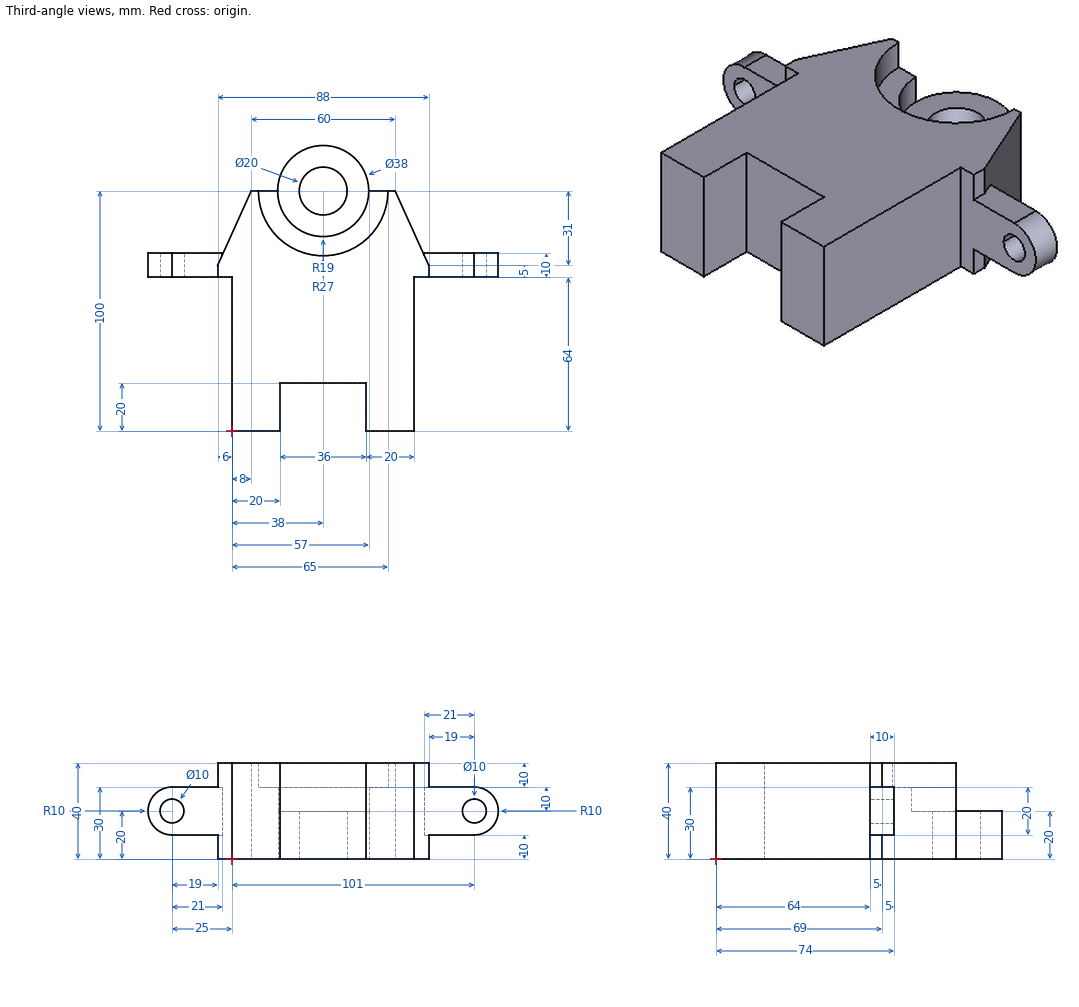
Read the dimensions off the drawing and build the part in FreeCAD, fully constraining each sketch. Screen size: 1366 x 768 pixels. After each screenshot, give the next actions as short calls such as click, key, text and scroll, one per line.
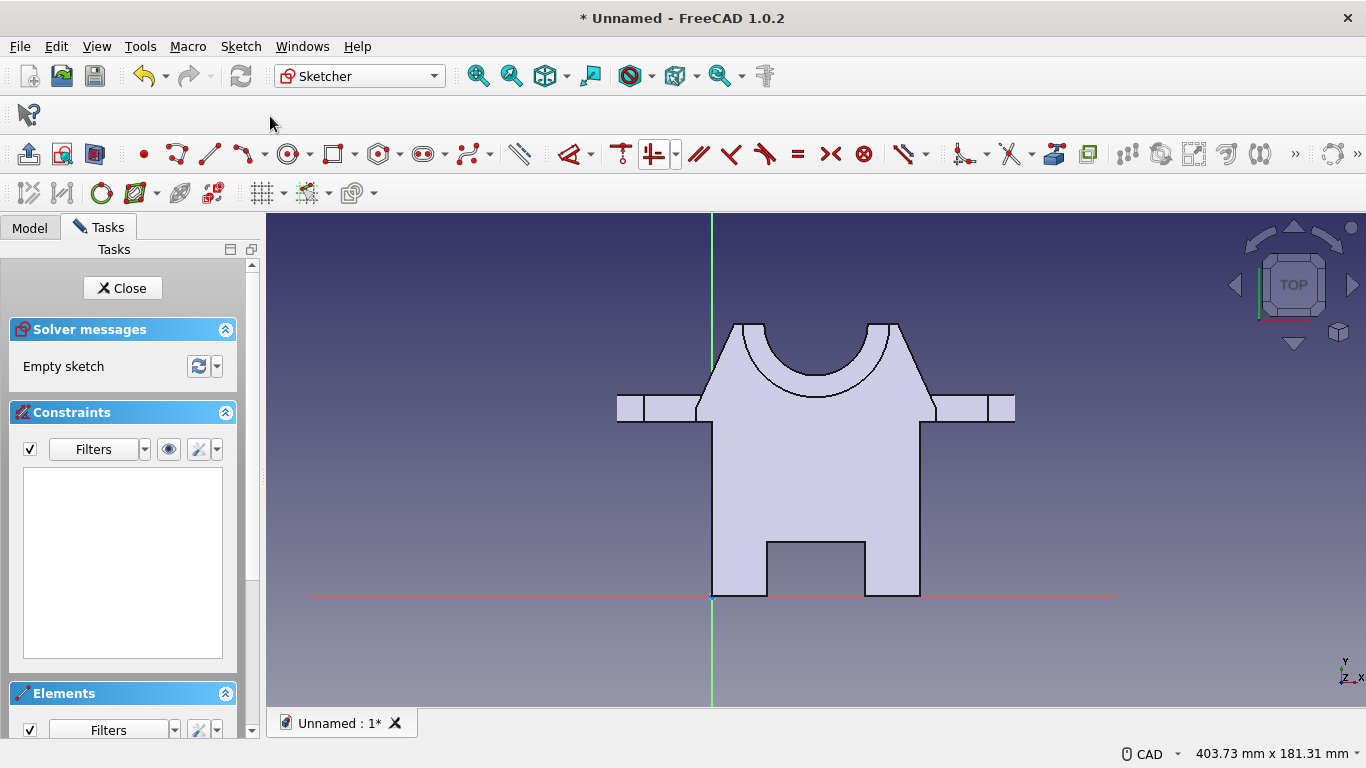
click(95, 154)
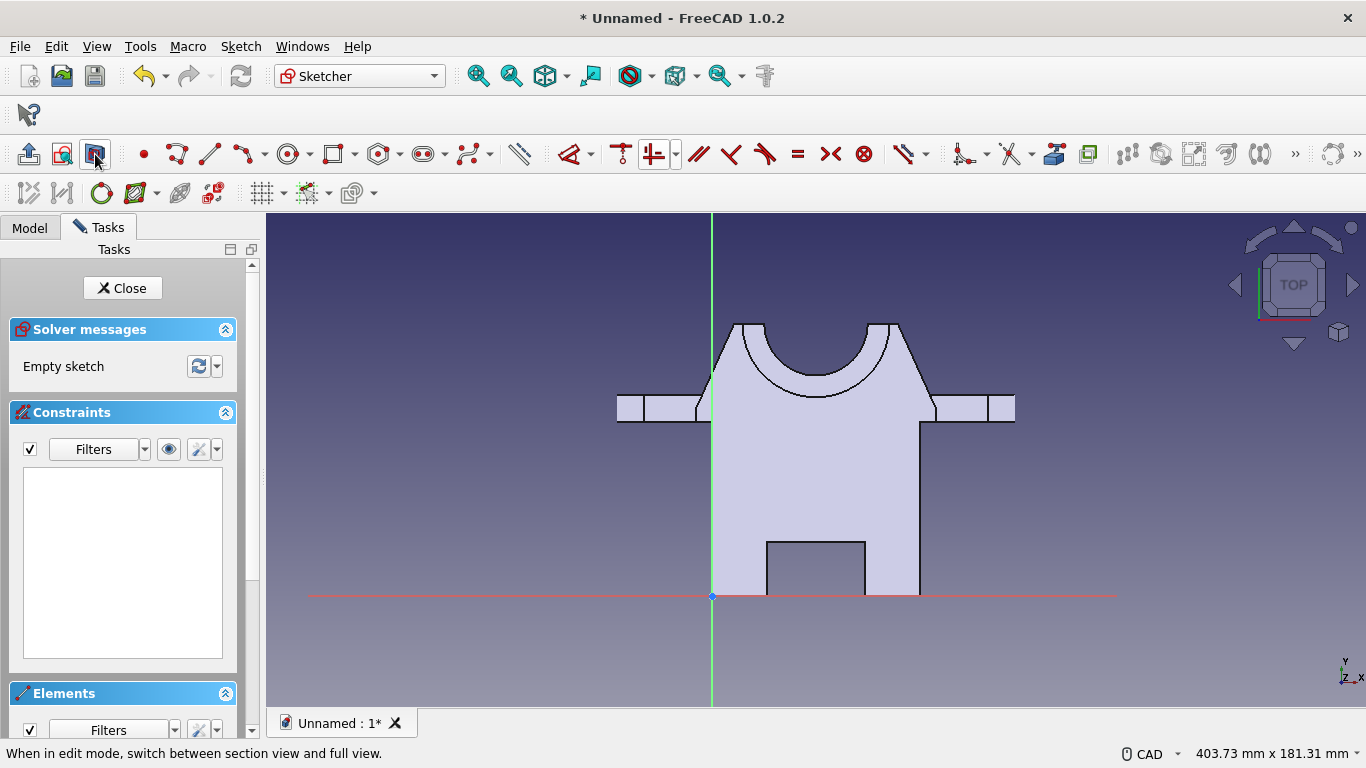
scroll(856, 244, up, 5)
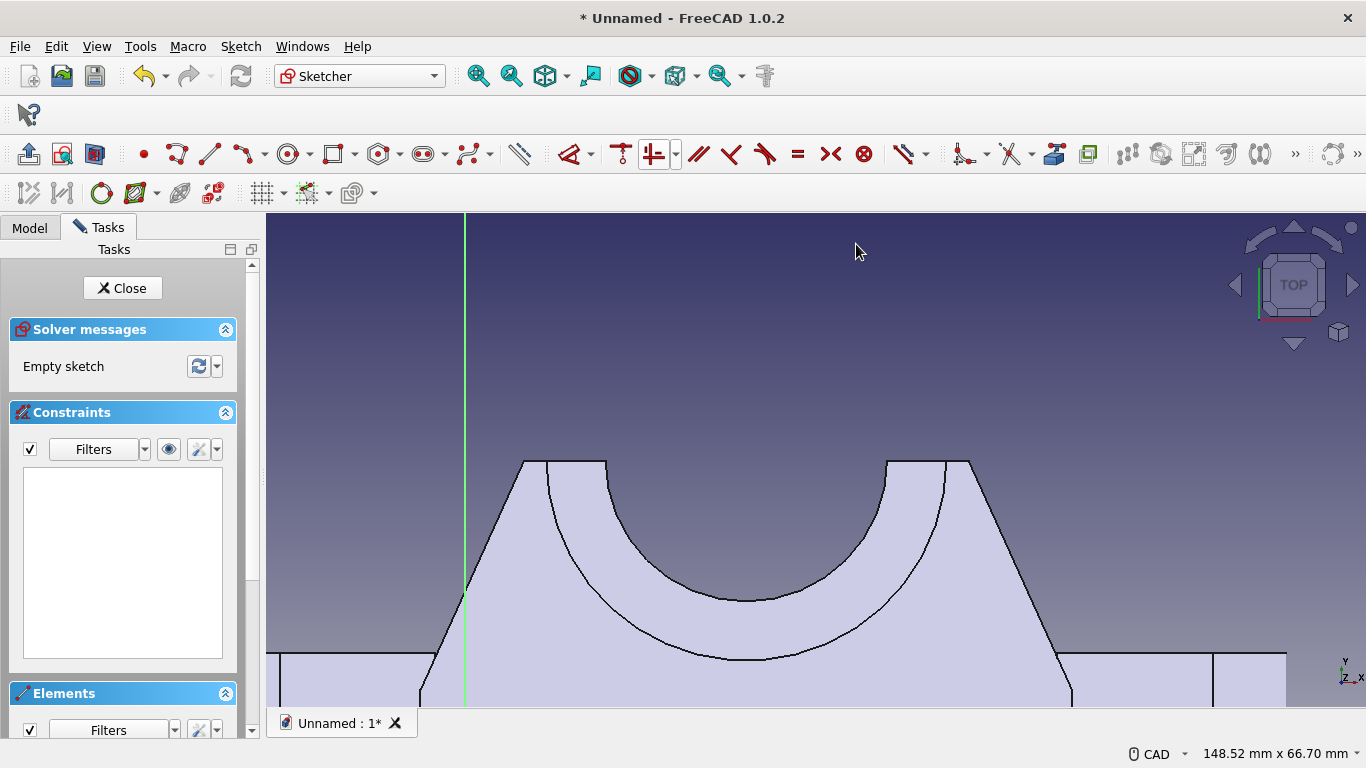
click(288, 154)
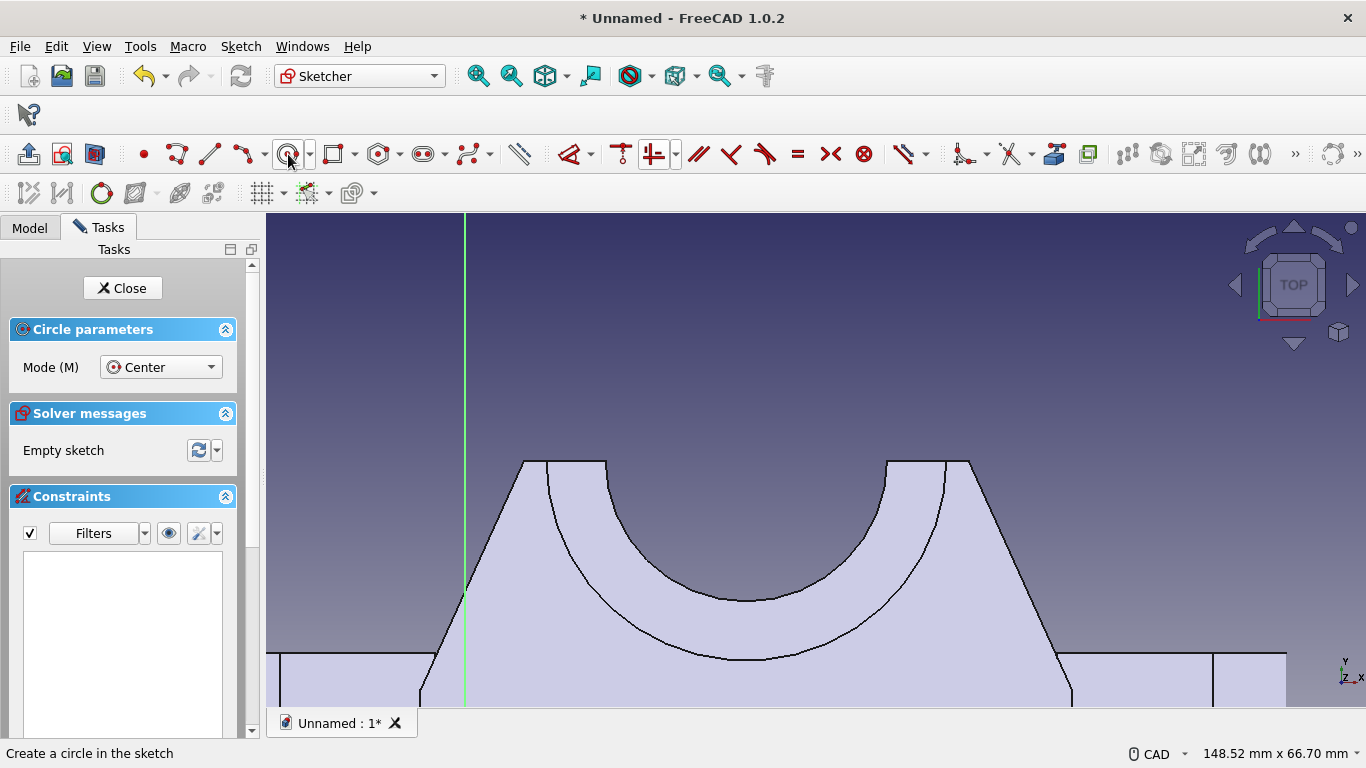
click(746, 461)
click(846, 361)
key(Escape)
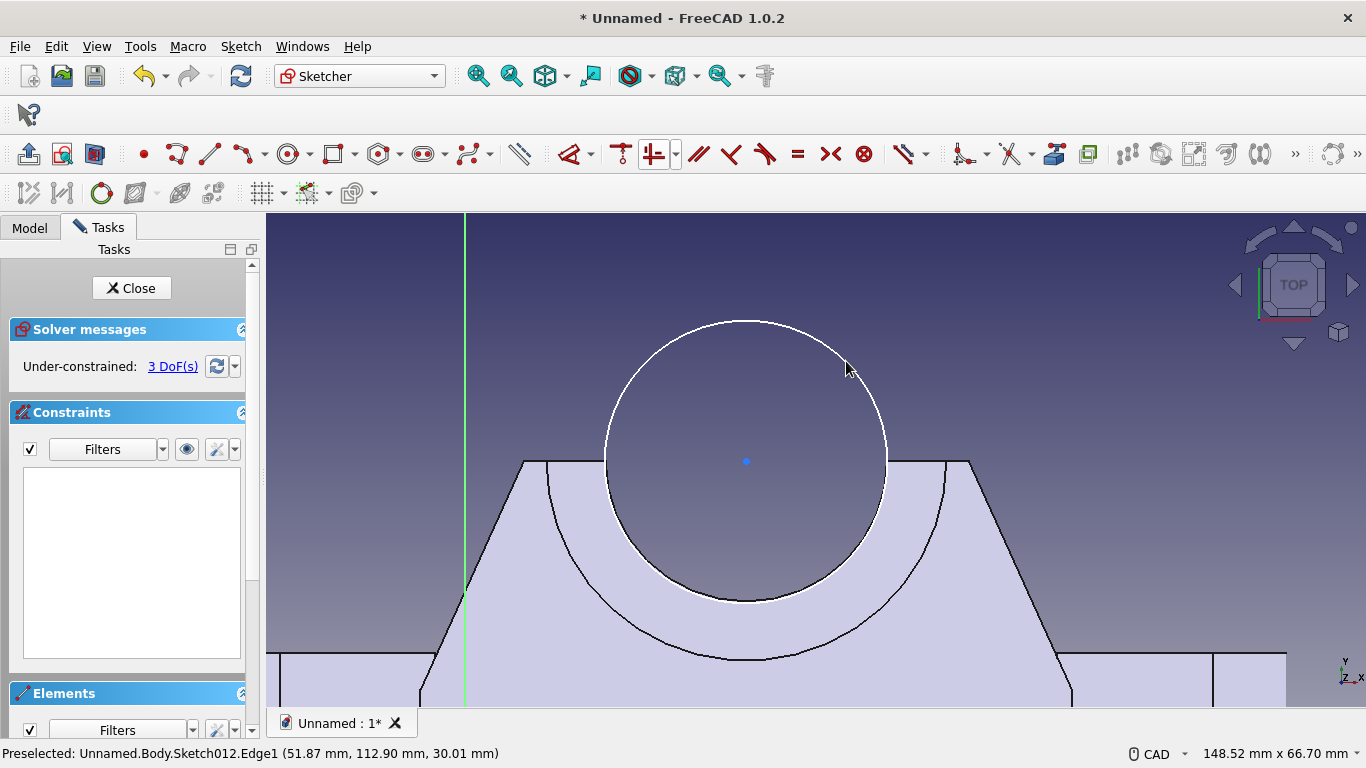
click(568, 154)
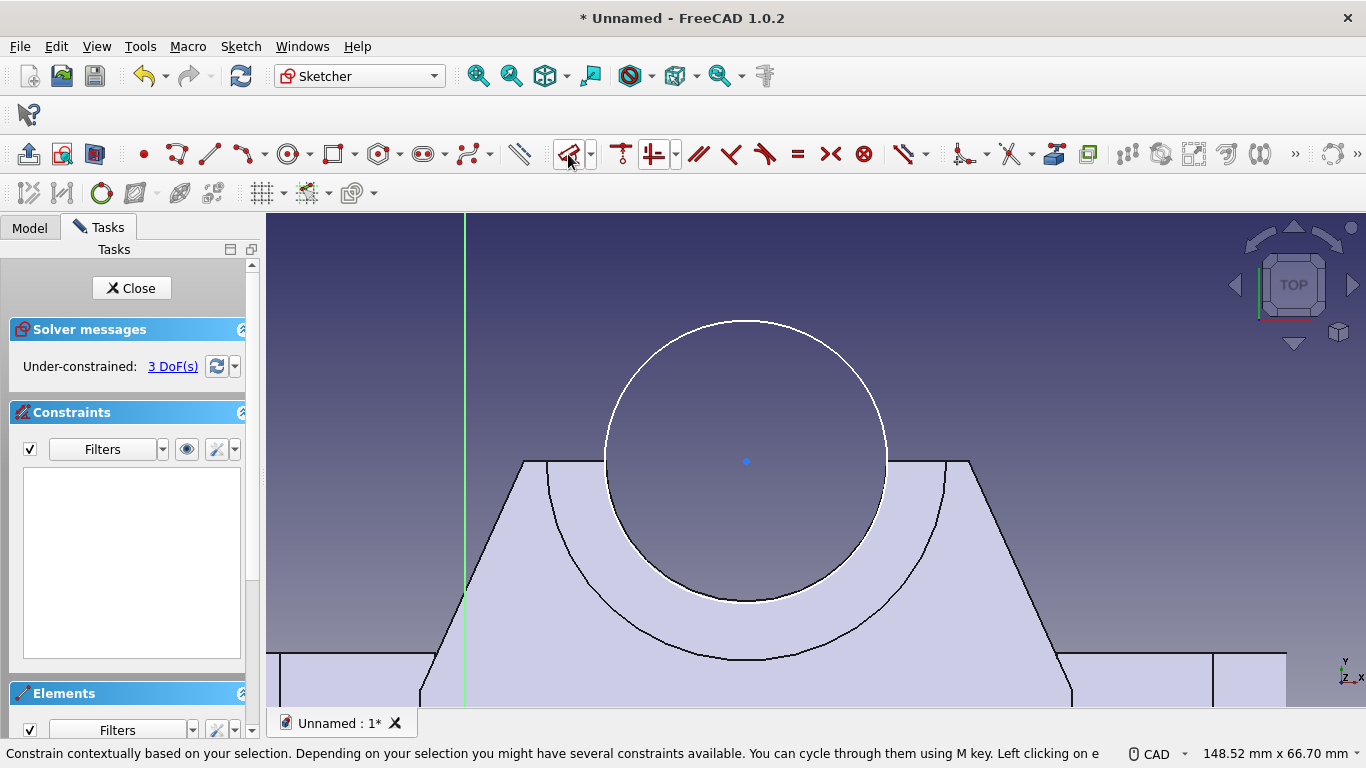
click(846, 362)
click(869, 339)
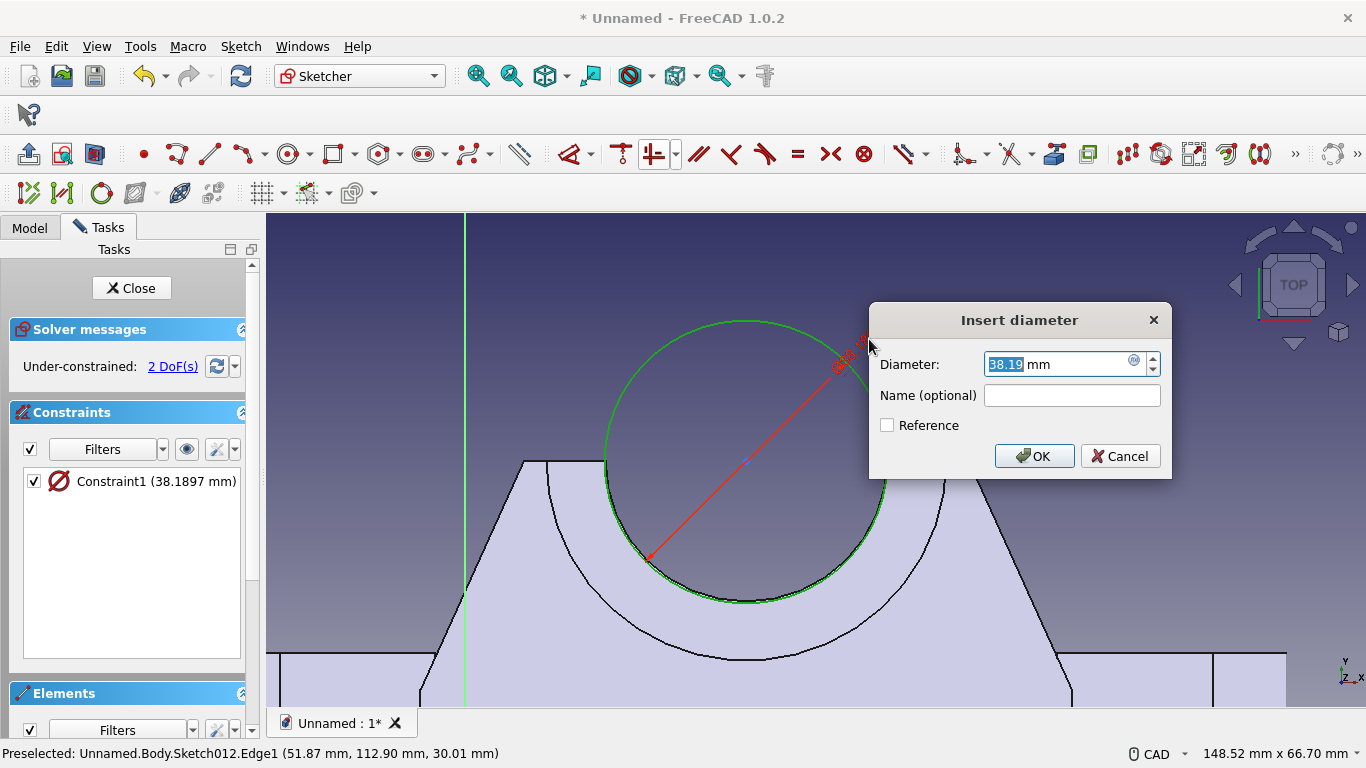
text(38)
key(Return)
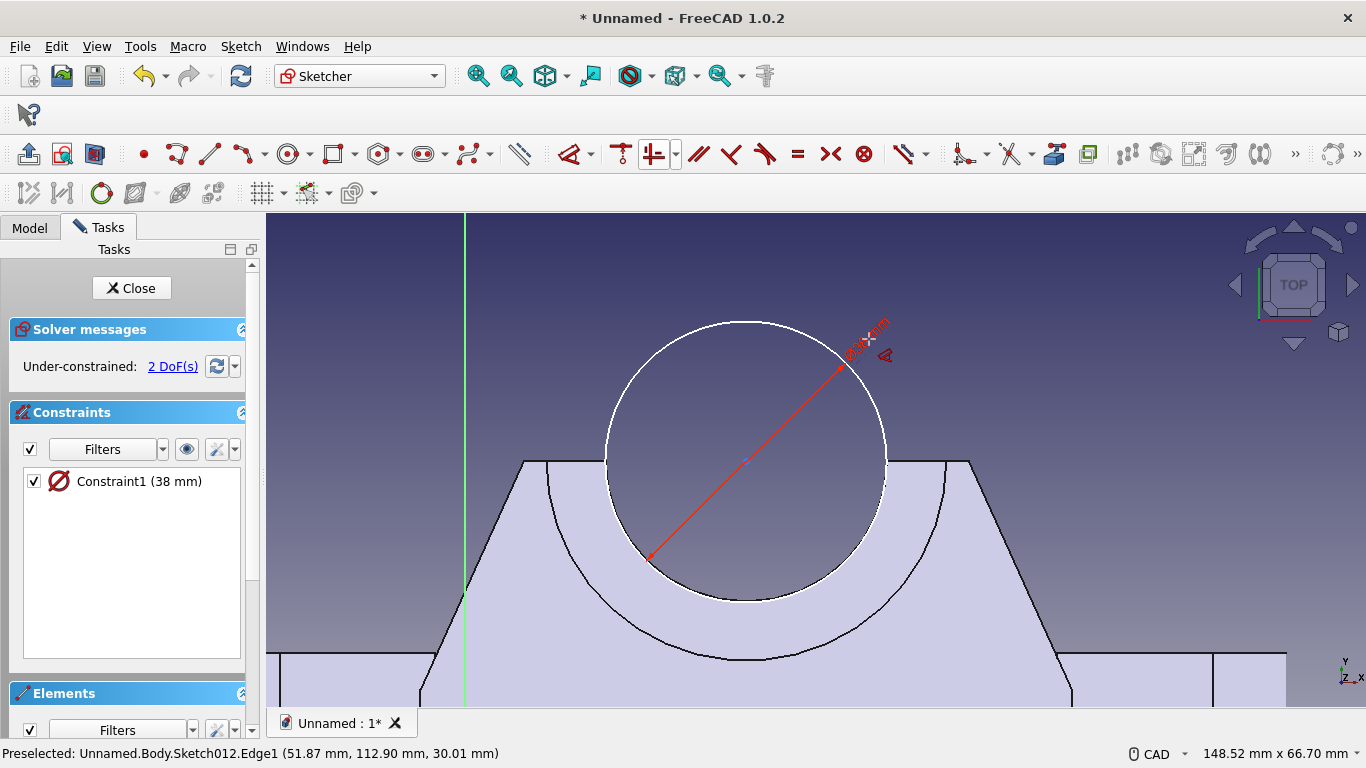
click(746, 462)
click(541, 428)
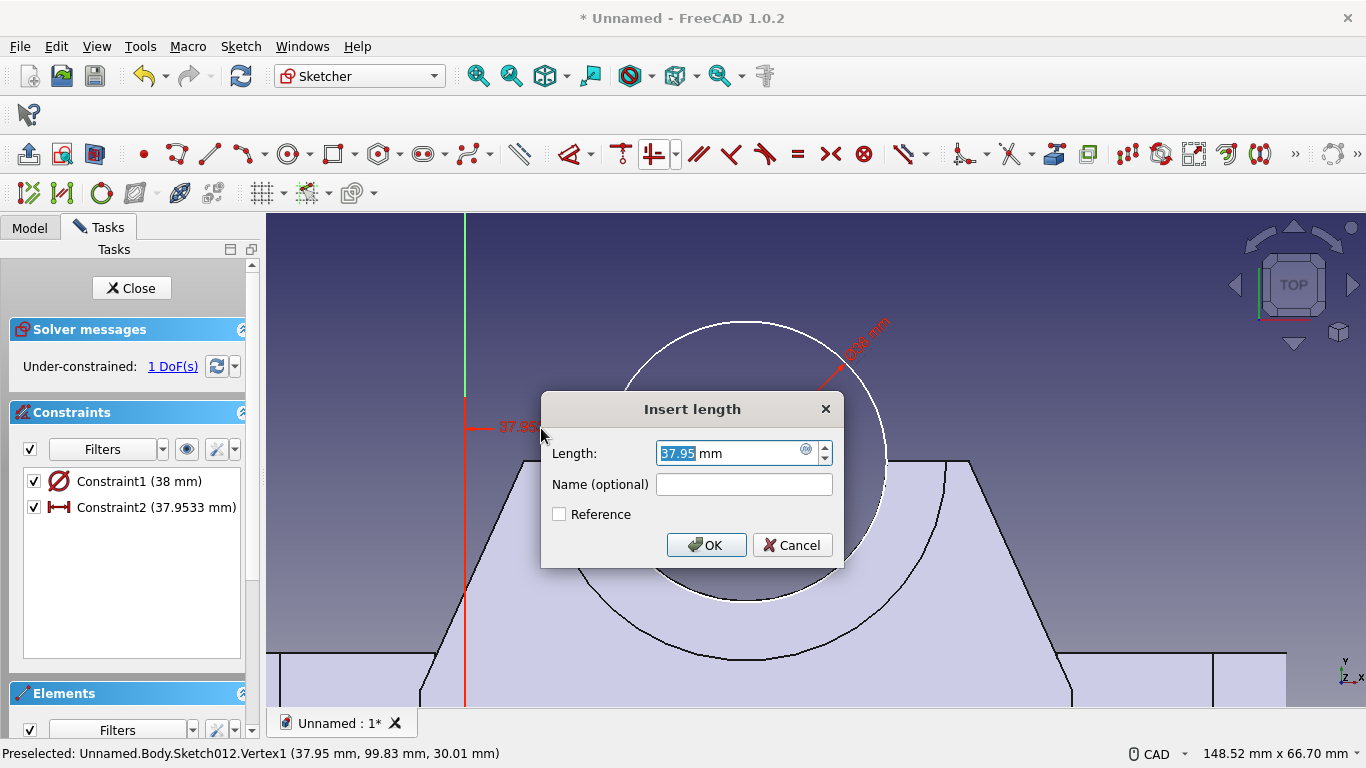
text(38)
key(Return)